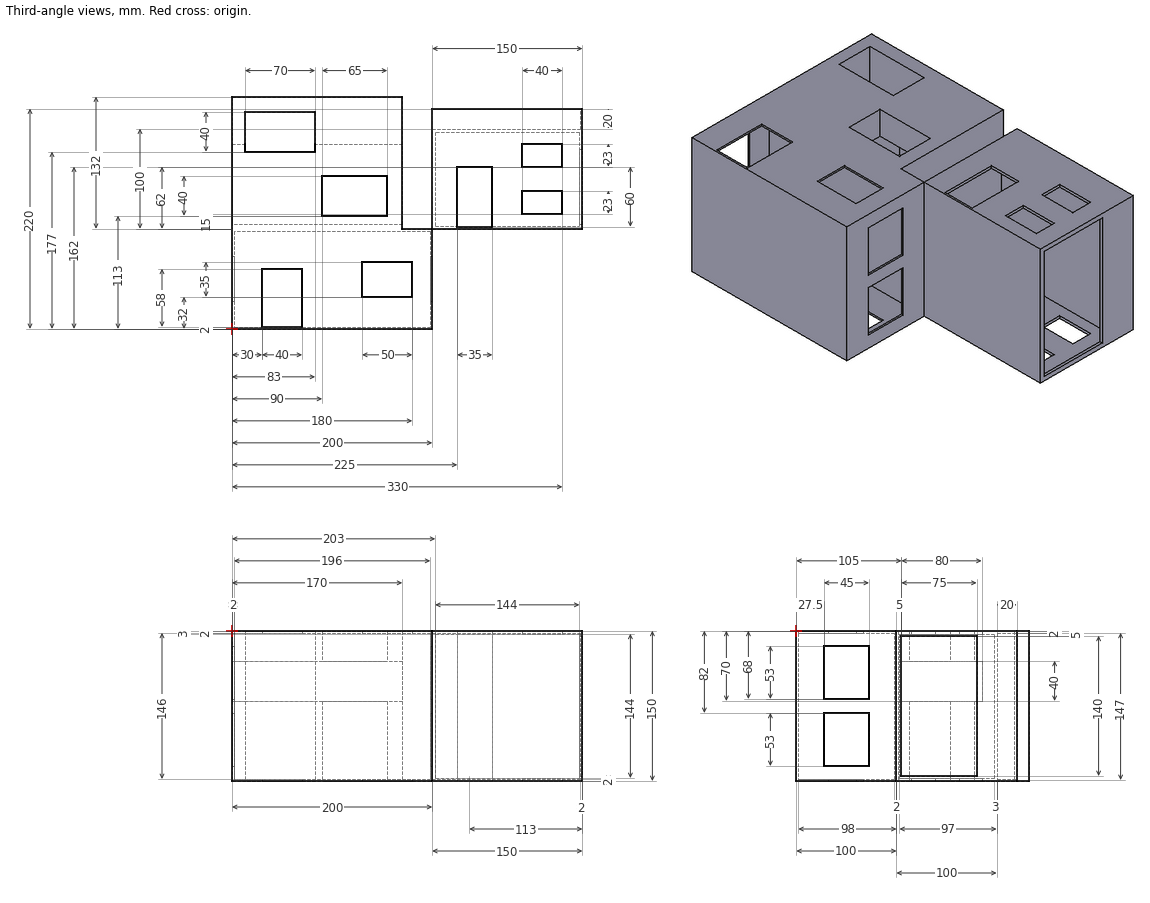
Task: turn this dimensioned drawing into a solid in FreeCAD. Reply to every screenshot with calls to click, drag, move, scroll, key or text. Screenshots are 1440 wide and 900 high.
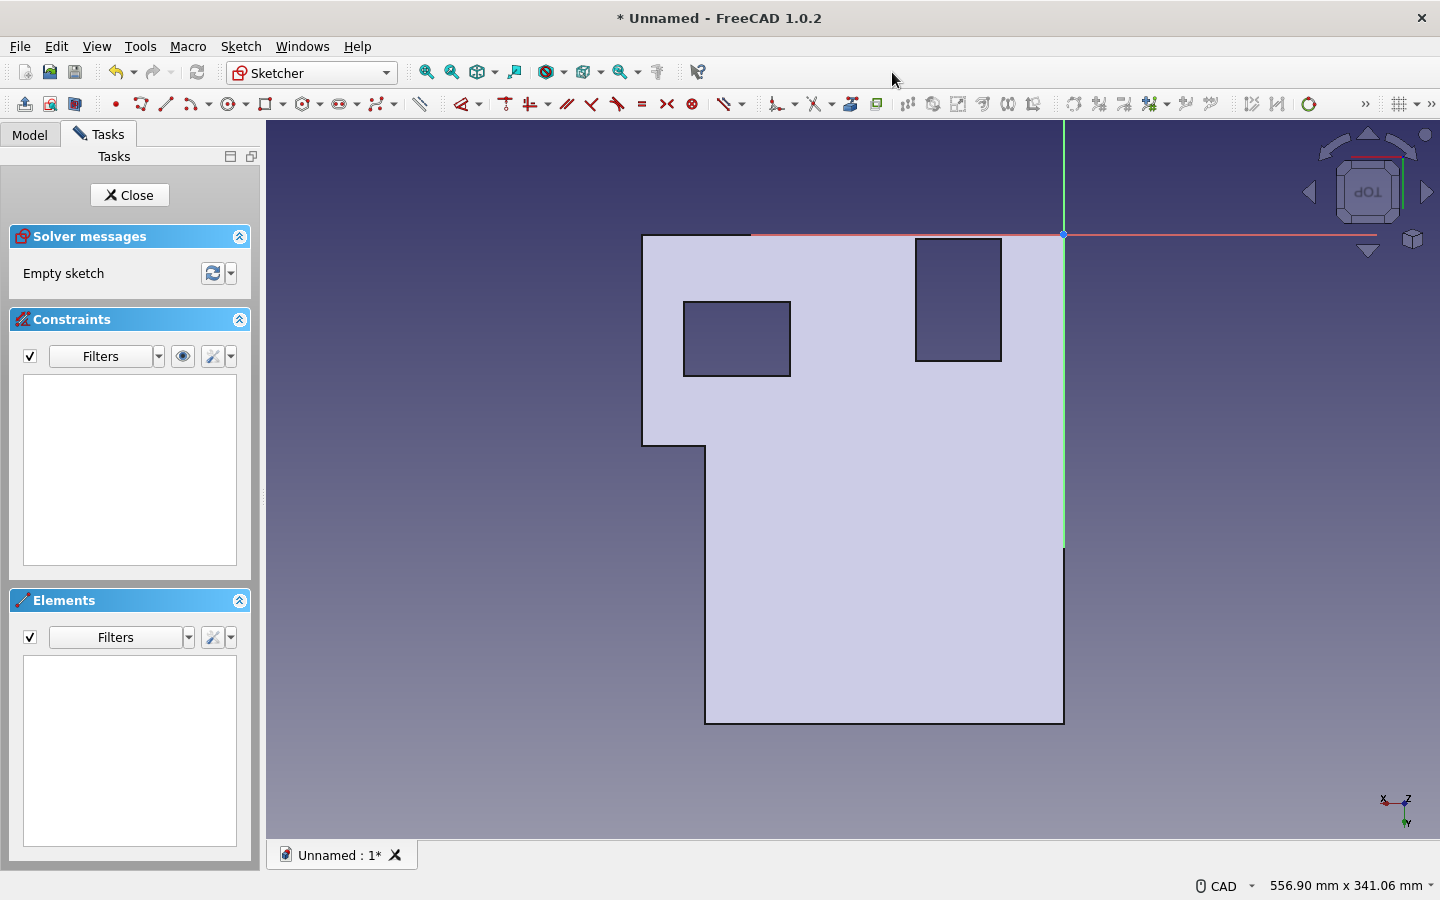
click(264, 104)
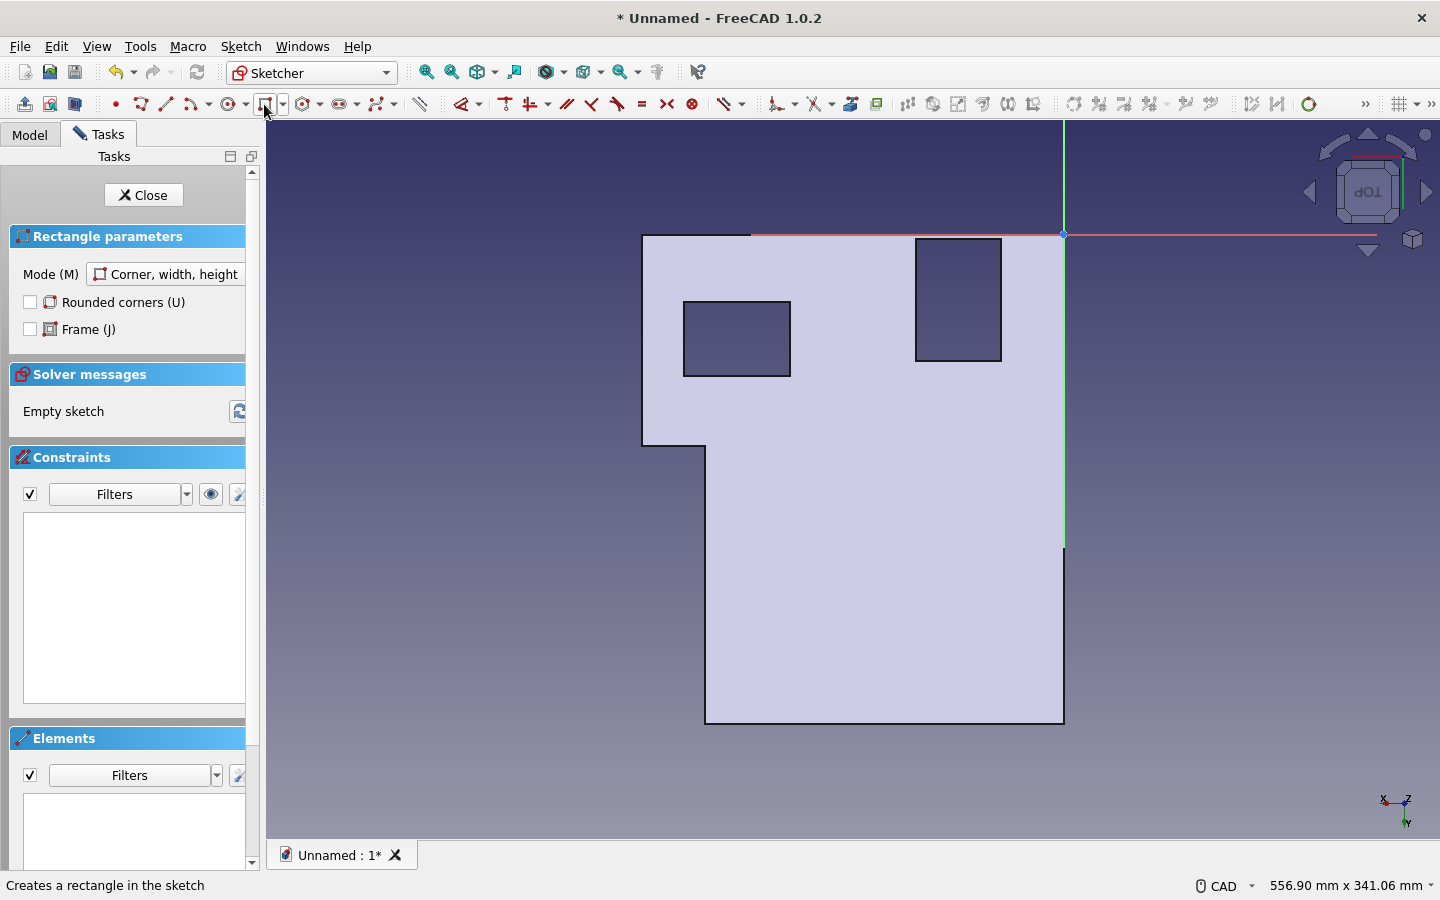
click(737, 473)
move(874, 558)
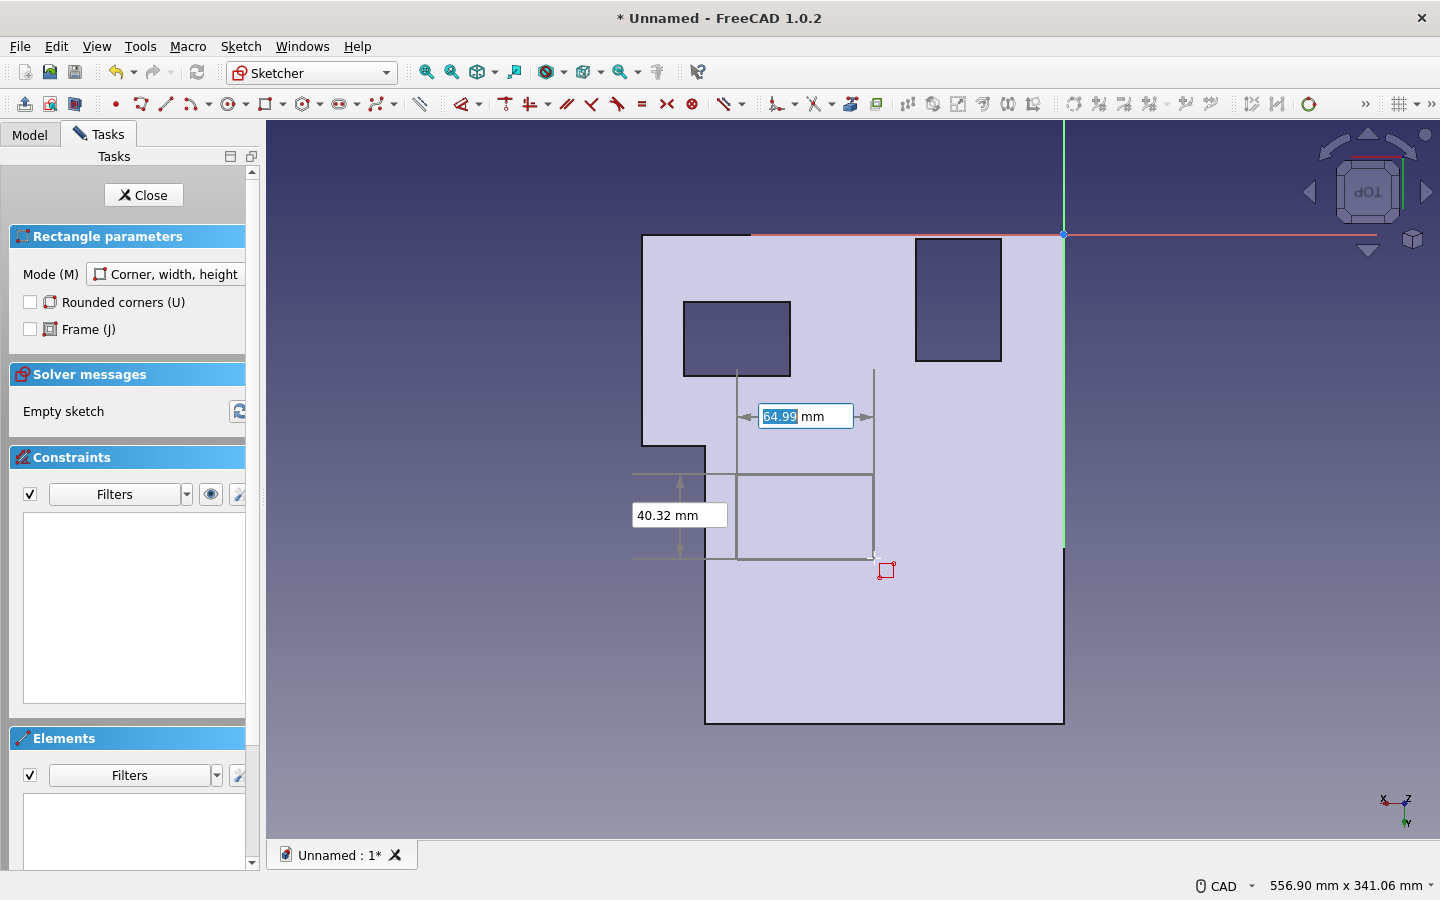
text(65)
key(Tab)
text(40)
key(Return)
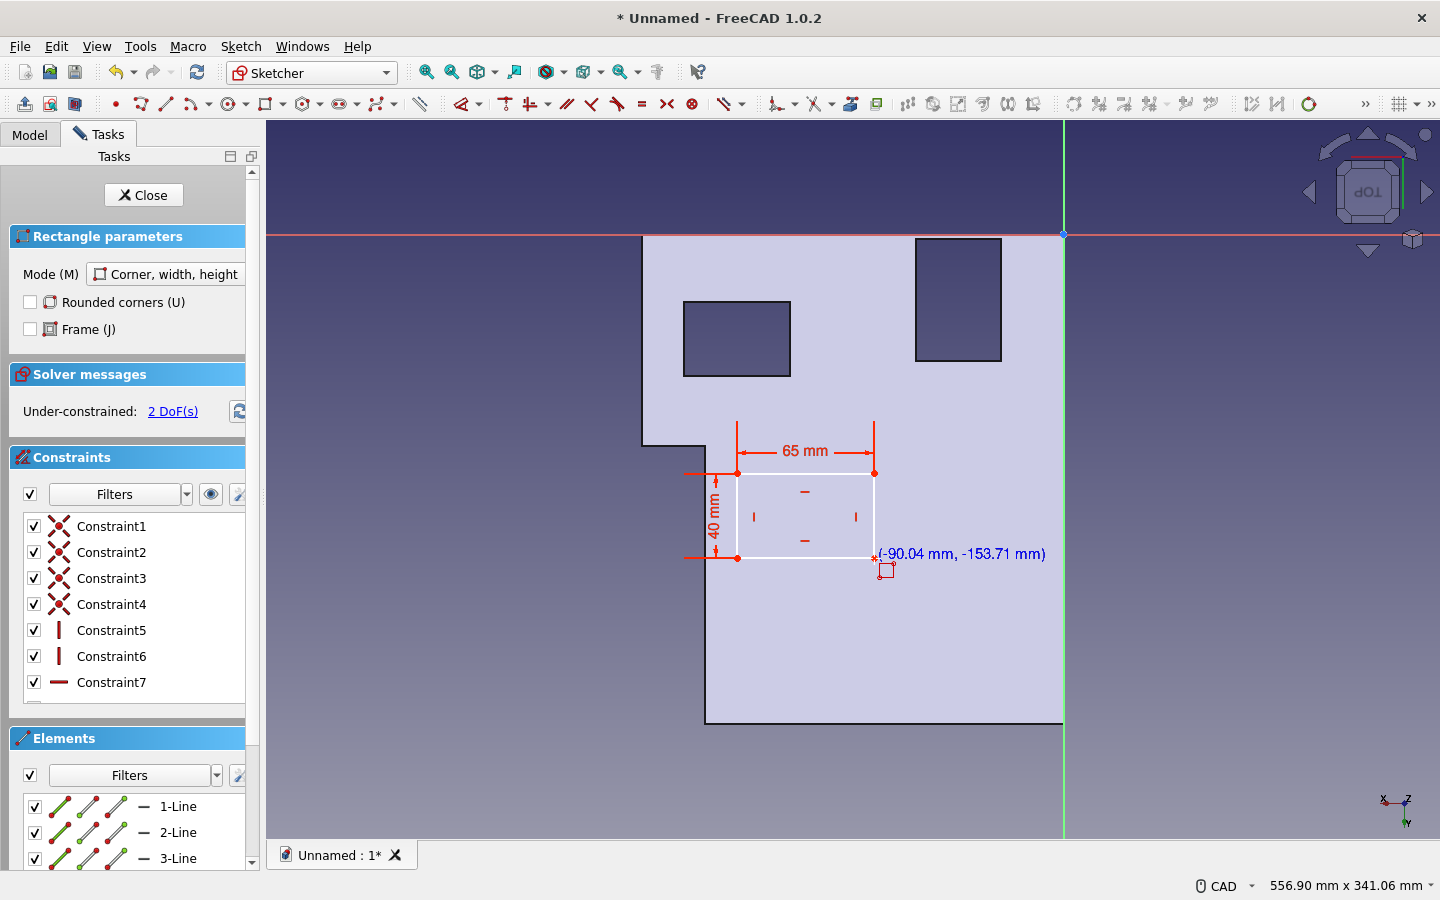
click(889, 608)
move(1036, 692)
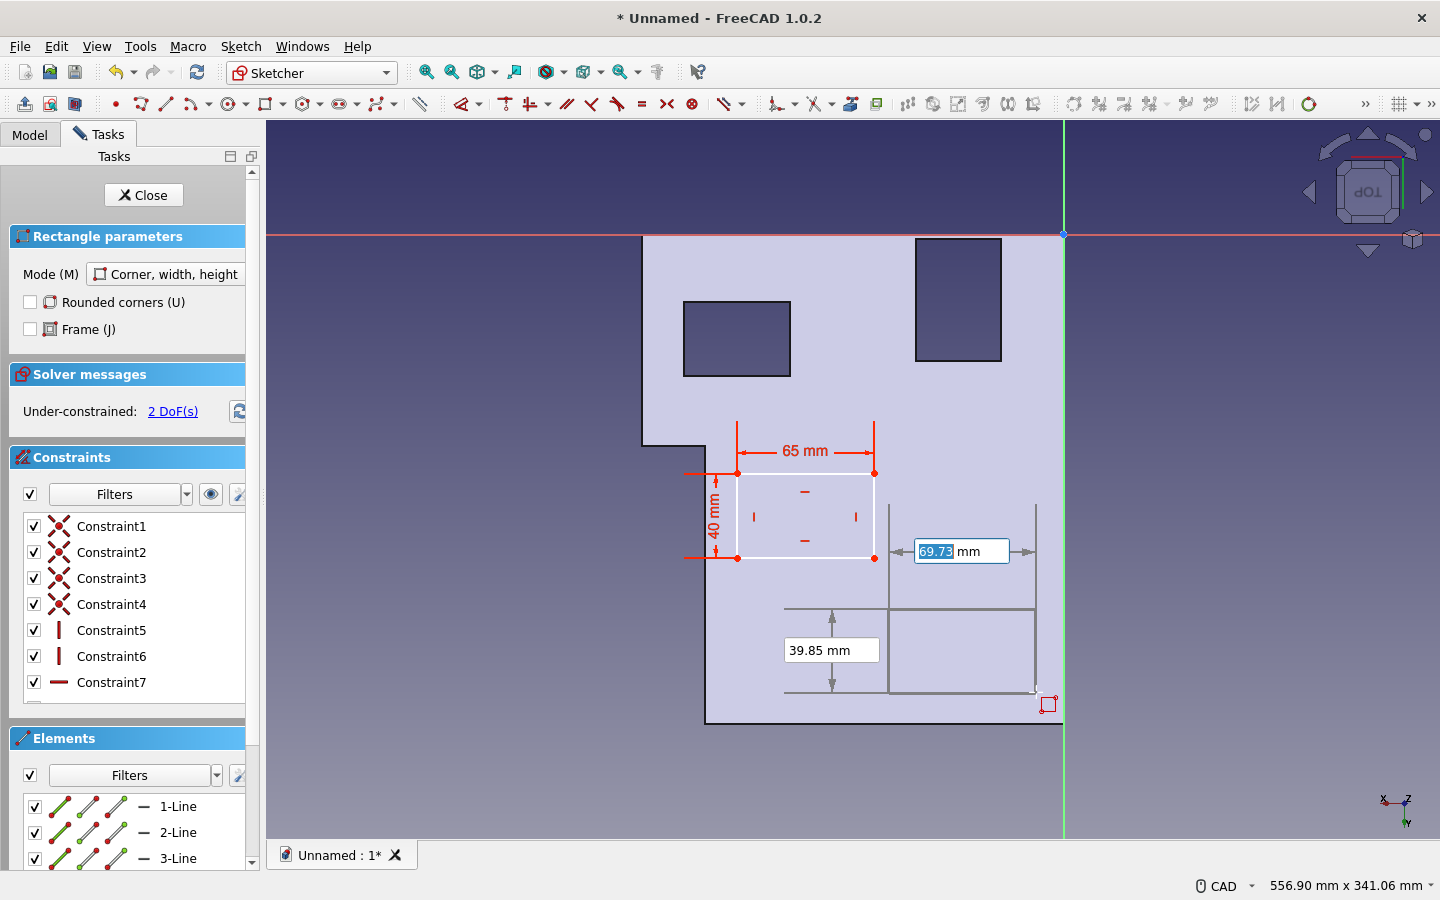
text(70)
key(Tab)
text(40)
key(Return)
key(Escape)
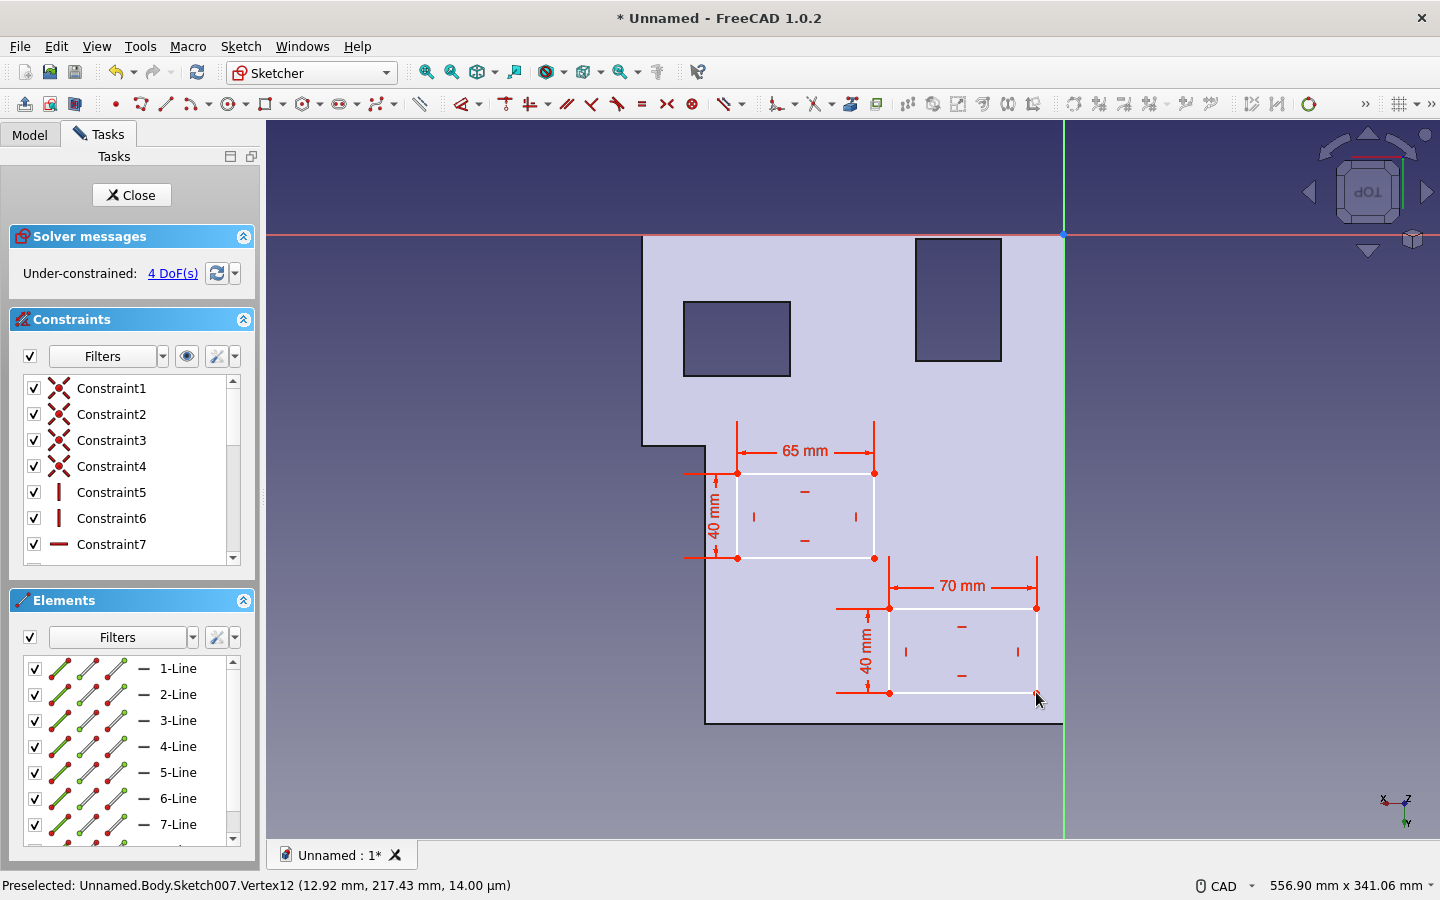
click(460, 104)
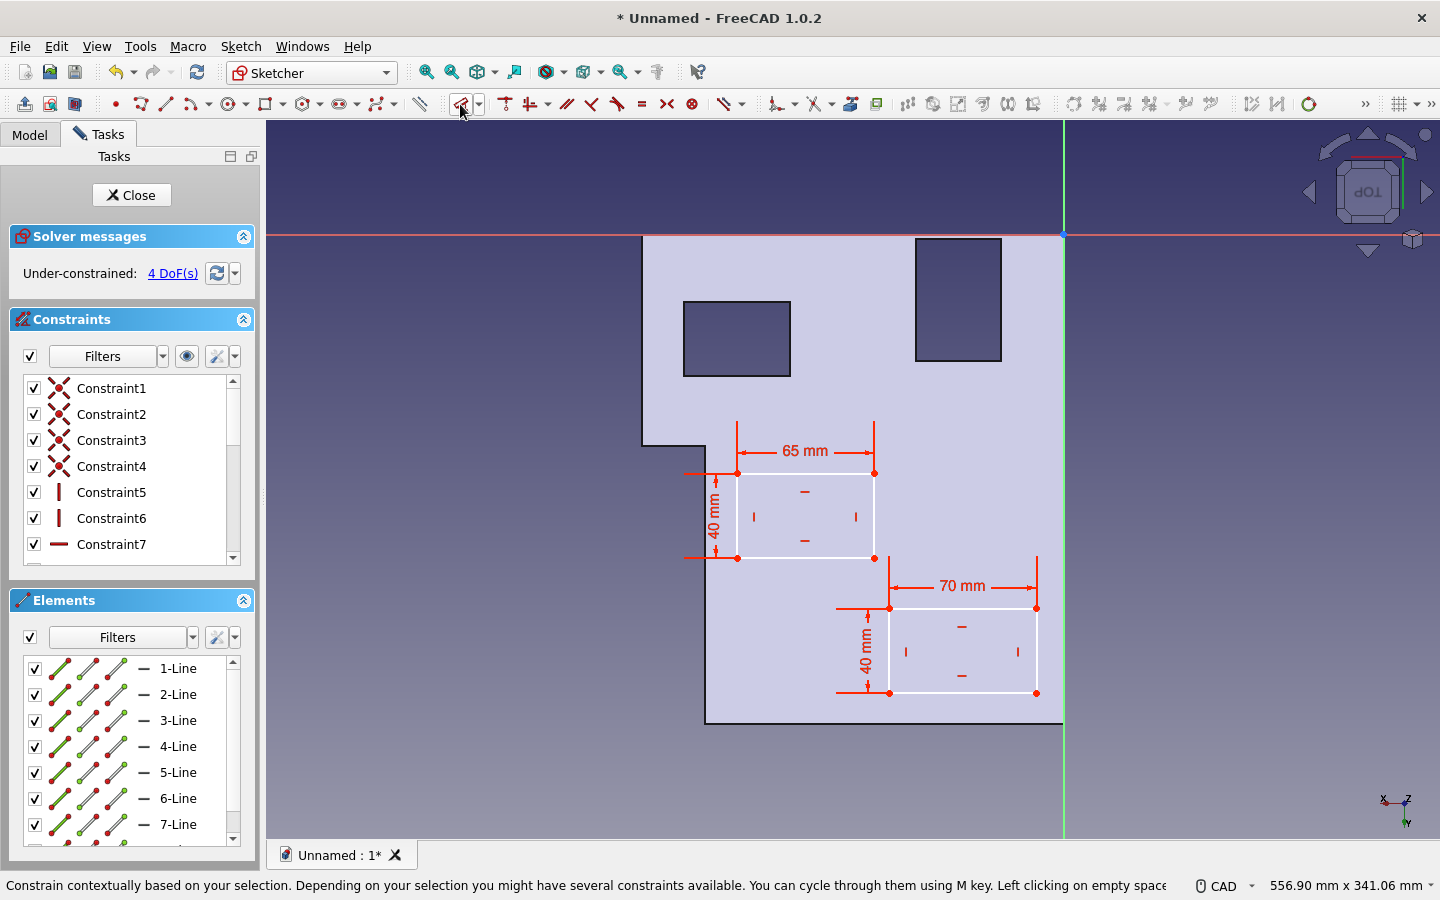
click(874, 558)
click(969, 201)